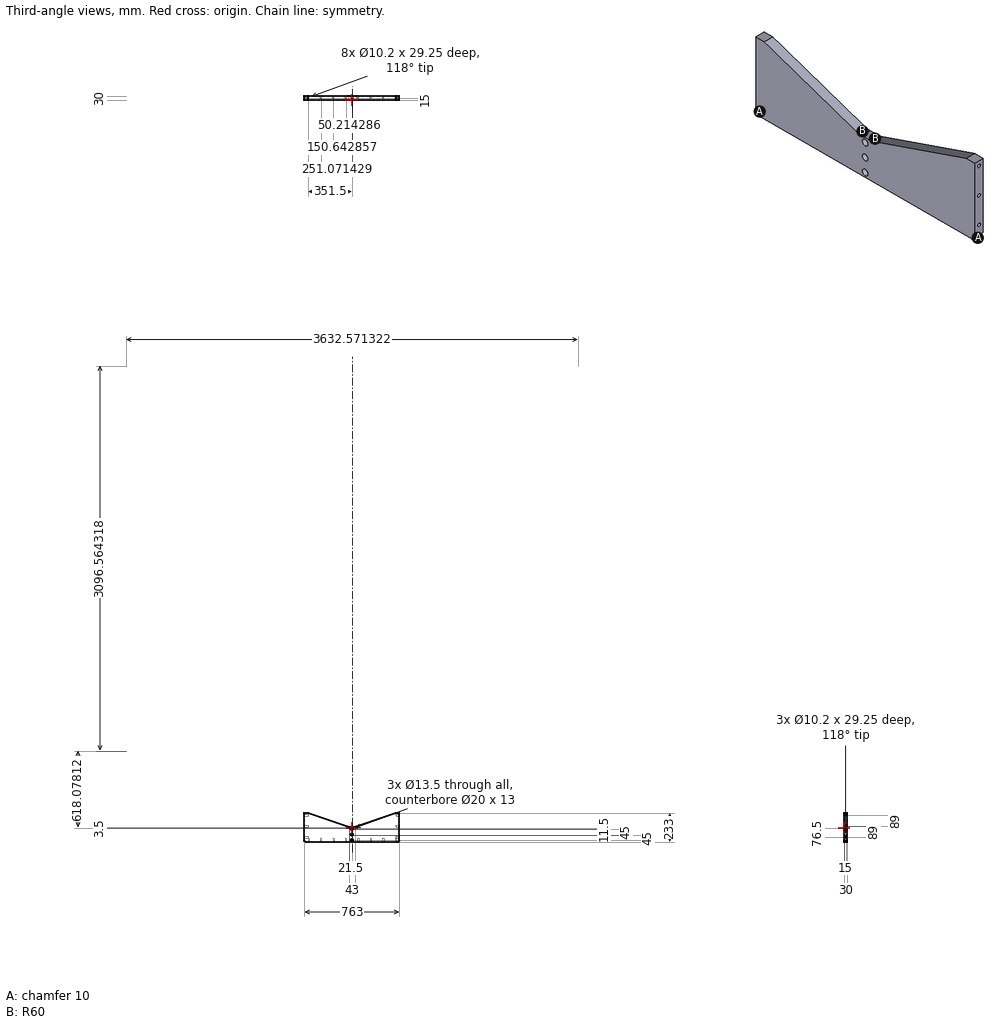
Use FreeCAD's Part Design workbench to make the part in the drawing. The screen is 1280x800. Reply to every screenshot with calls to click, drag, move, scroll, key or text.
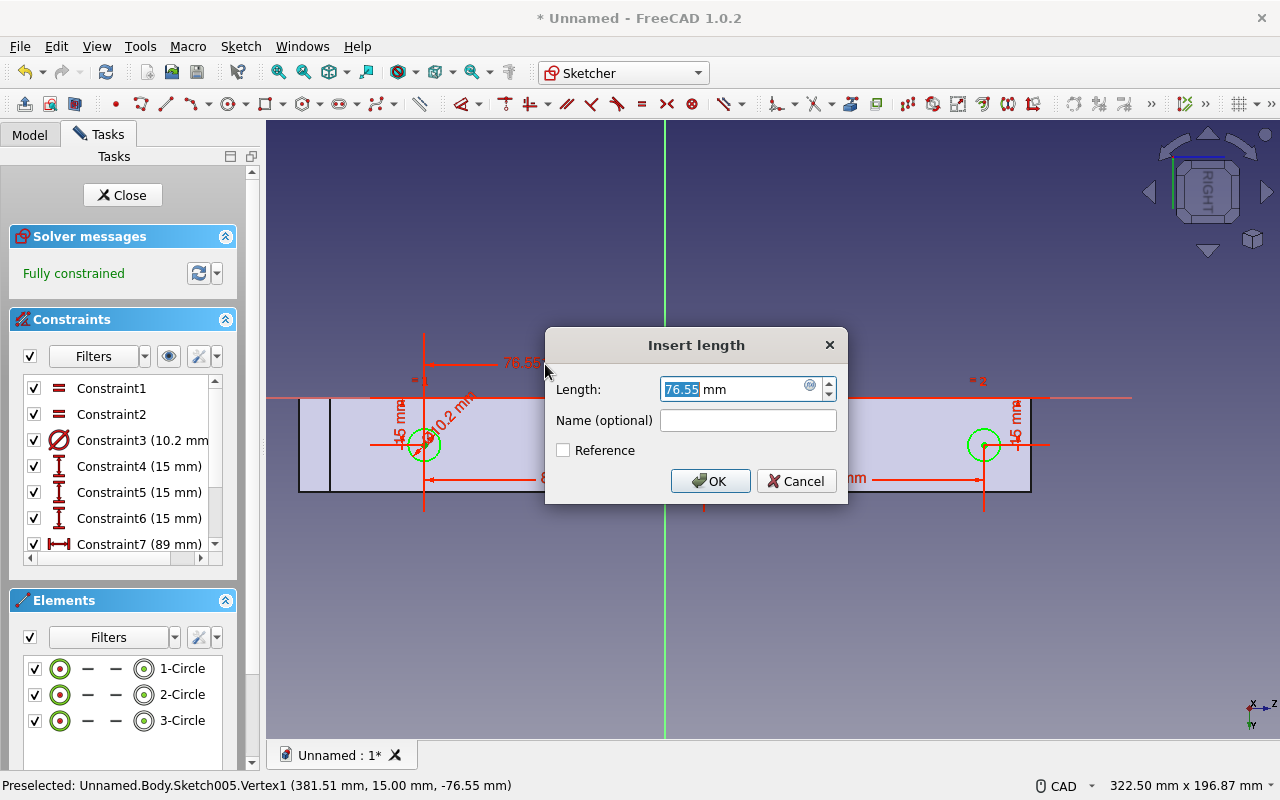
text(76.5)
key(Return)
key(Escape)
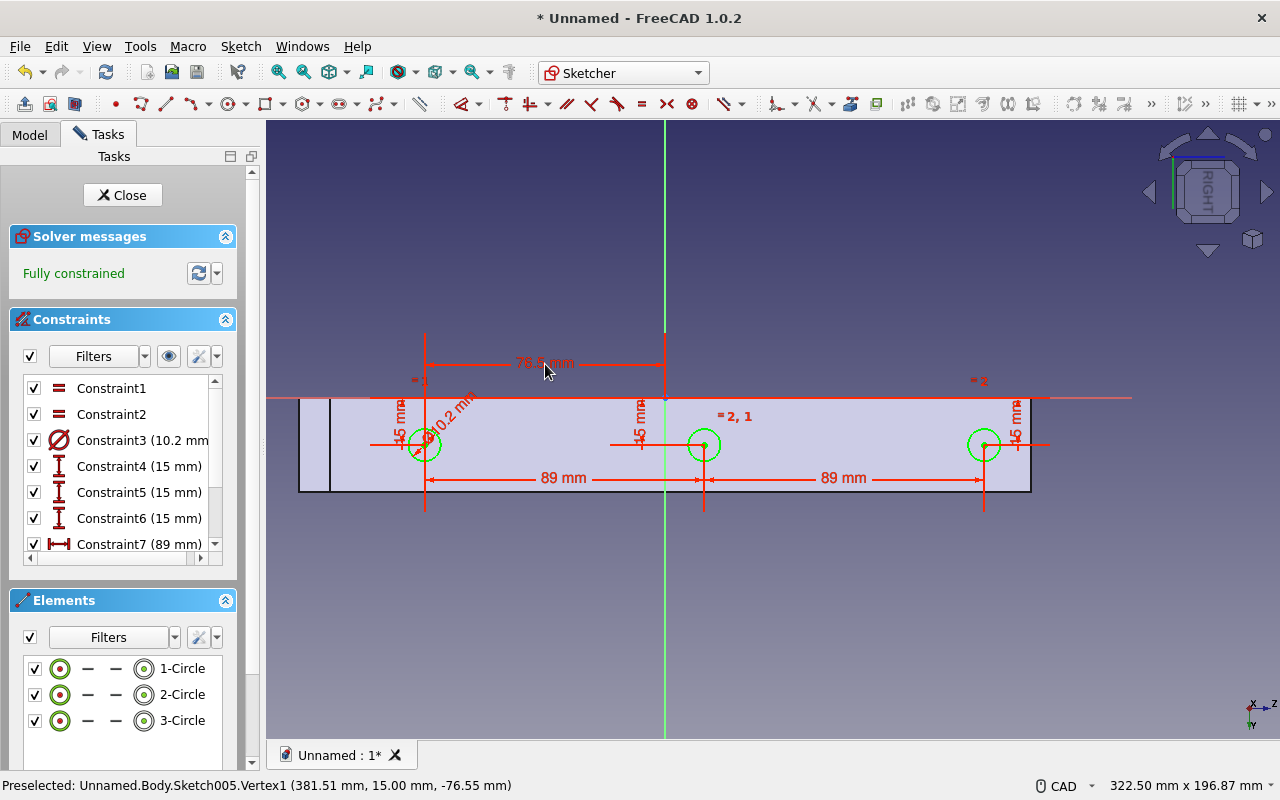
click(123, 195)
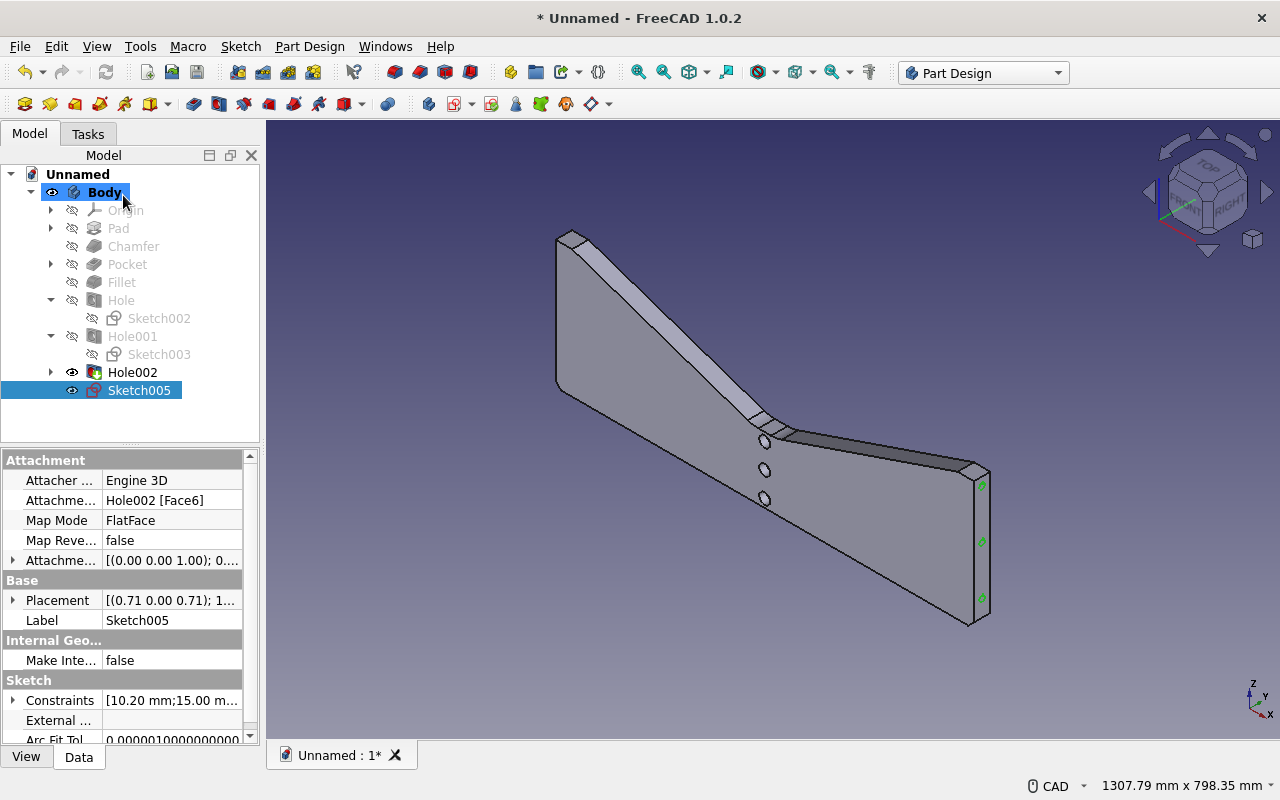
click(219, 104)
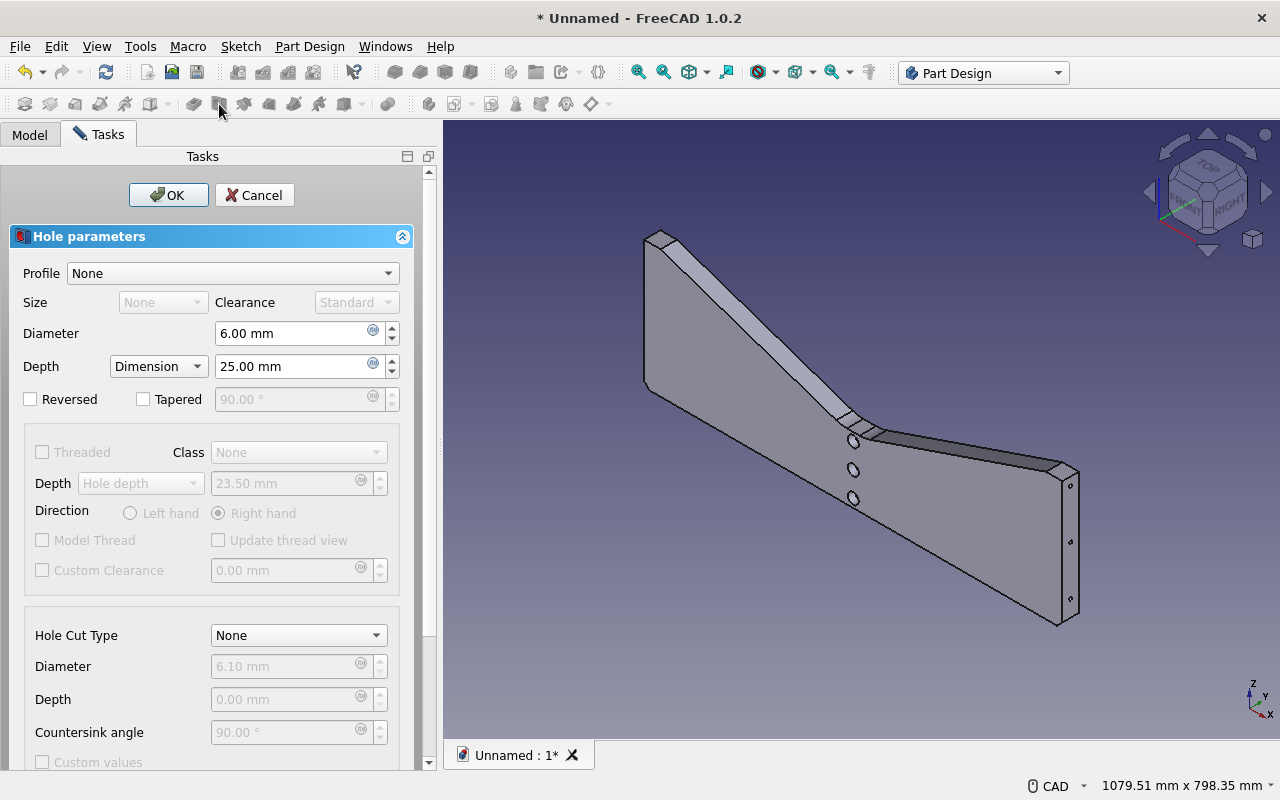
triple_click(300, 334)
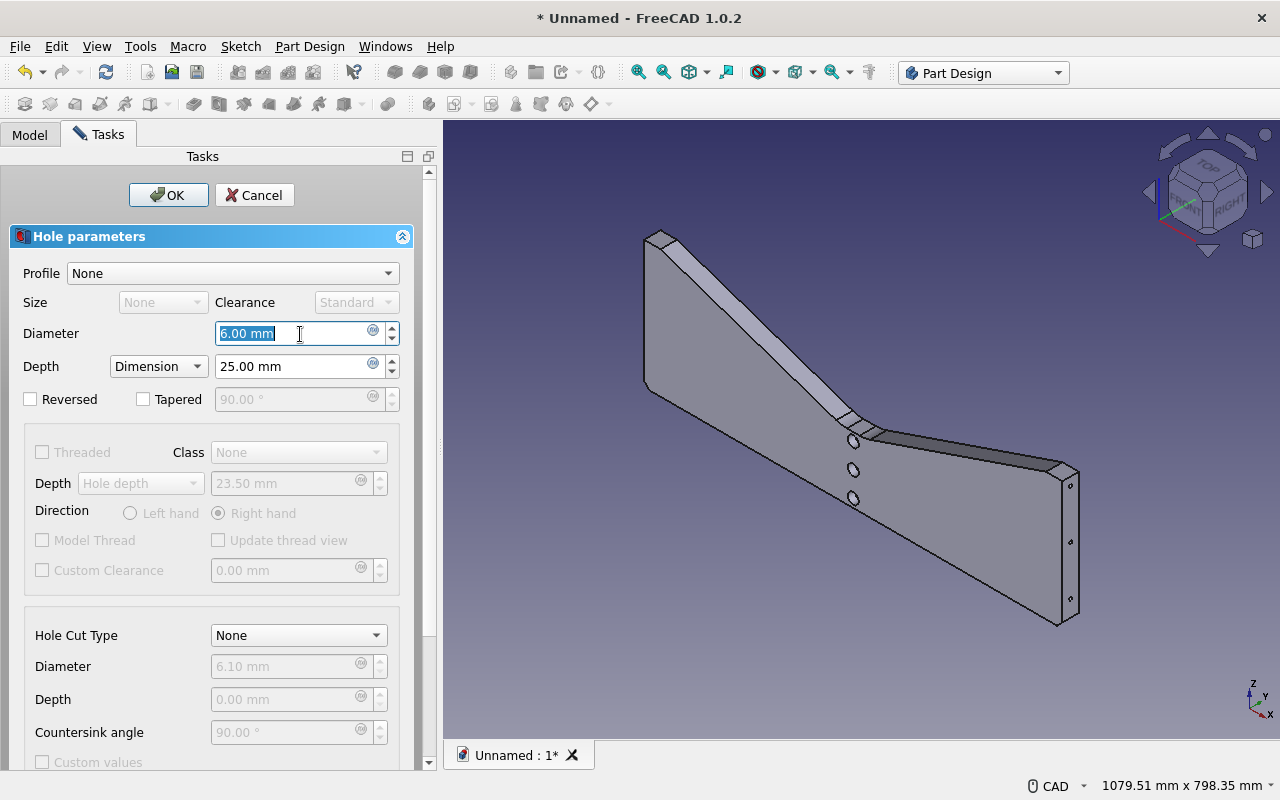
text(10.2)
key(Tab)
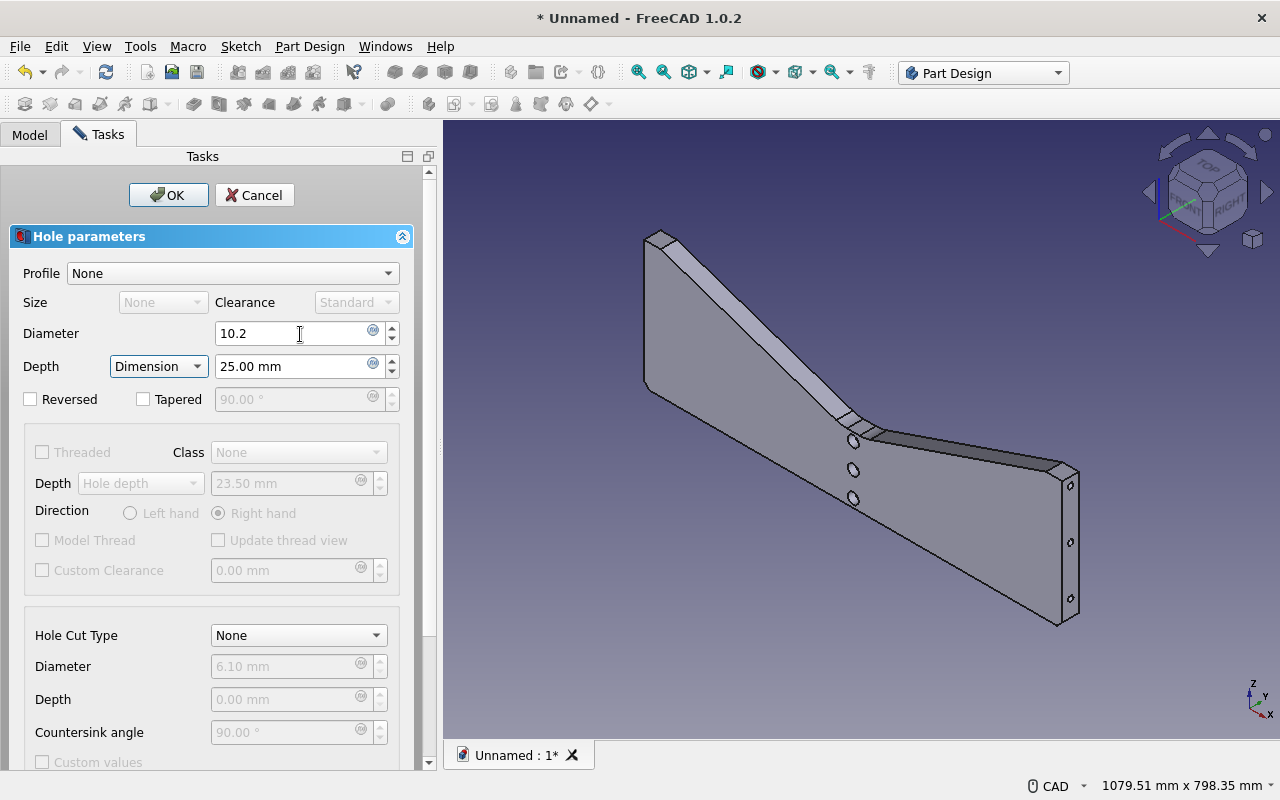
triple_click(300, 366)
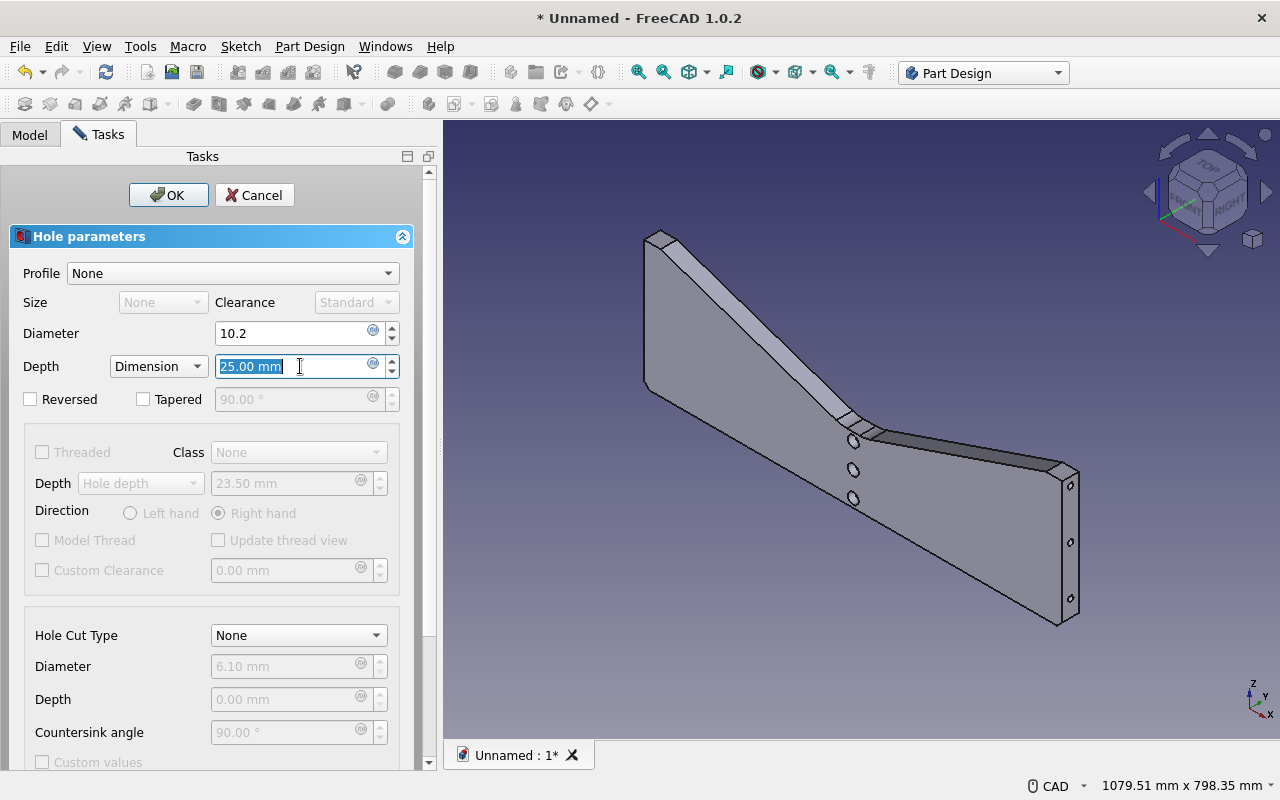
text(29.25)
key(Tab)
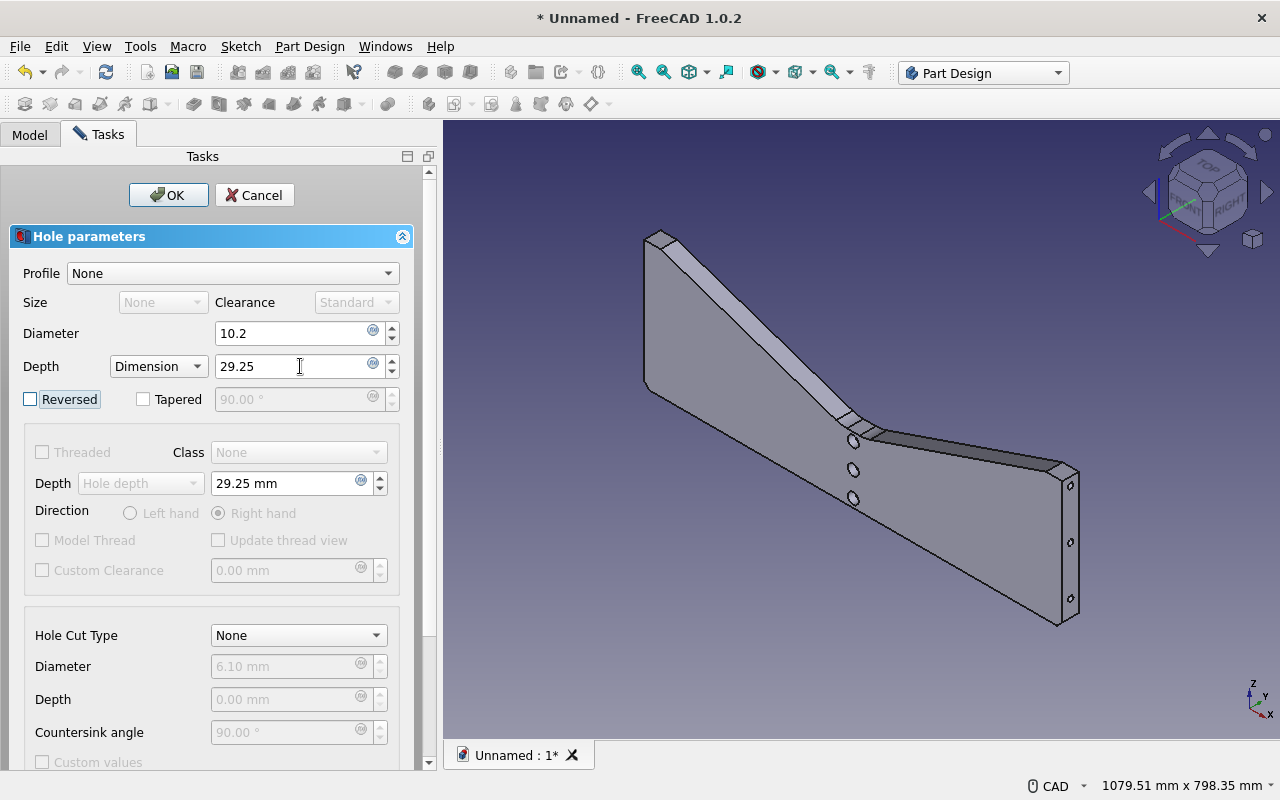
click(169, 195)